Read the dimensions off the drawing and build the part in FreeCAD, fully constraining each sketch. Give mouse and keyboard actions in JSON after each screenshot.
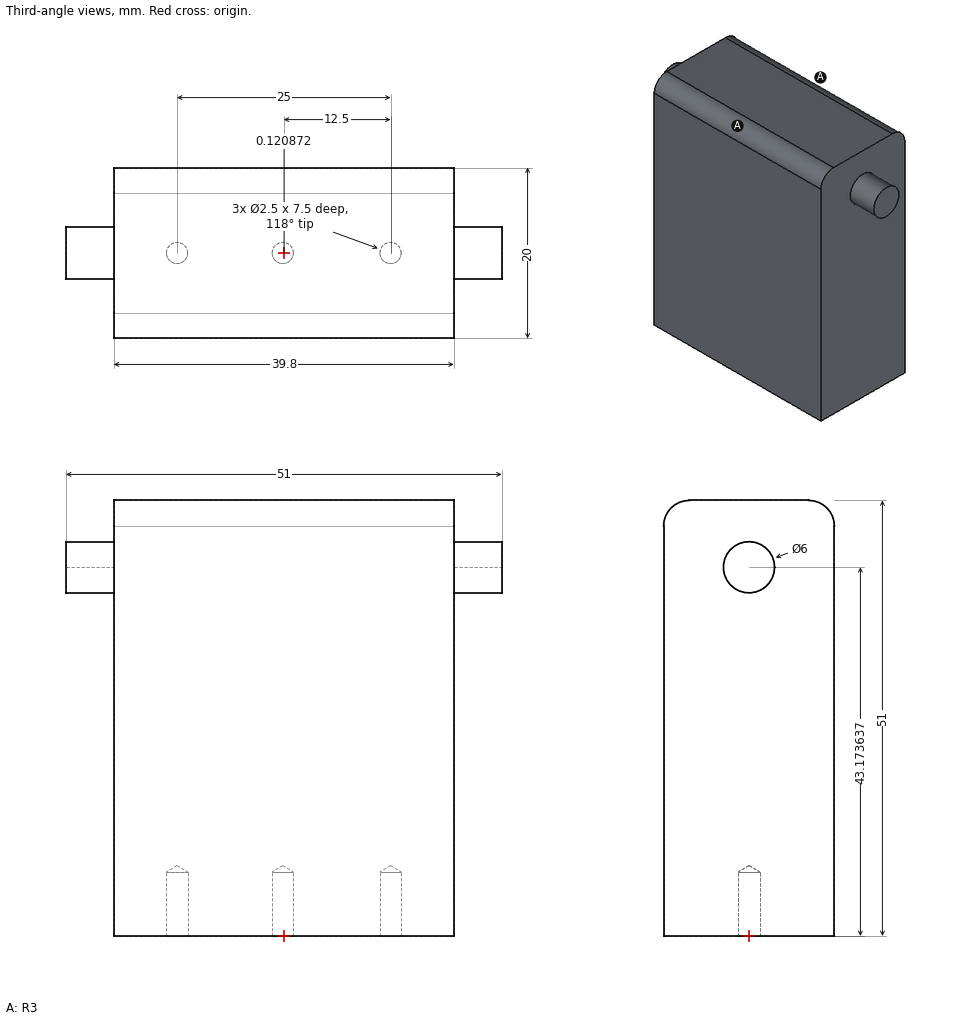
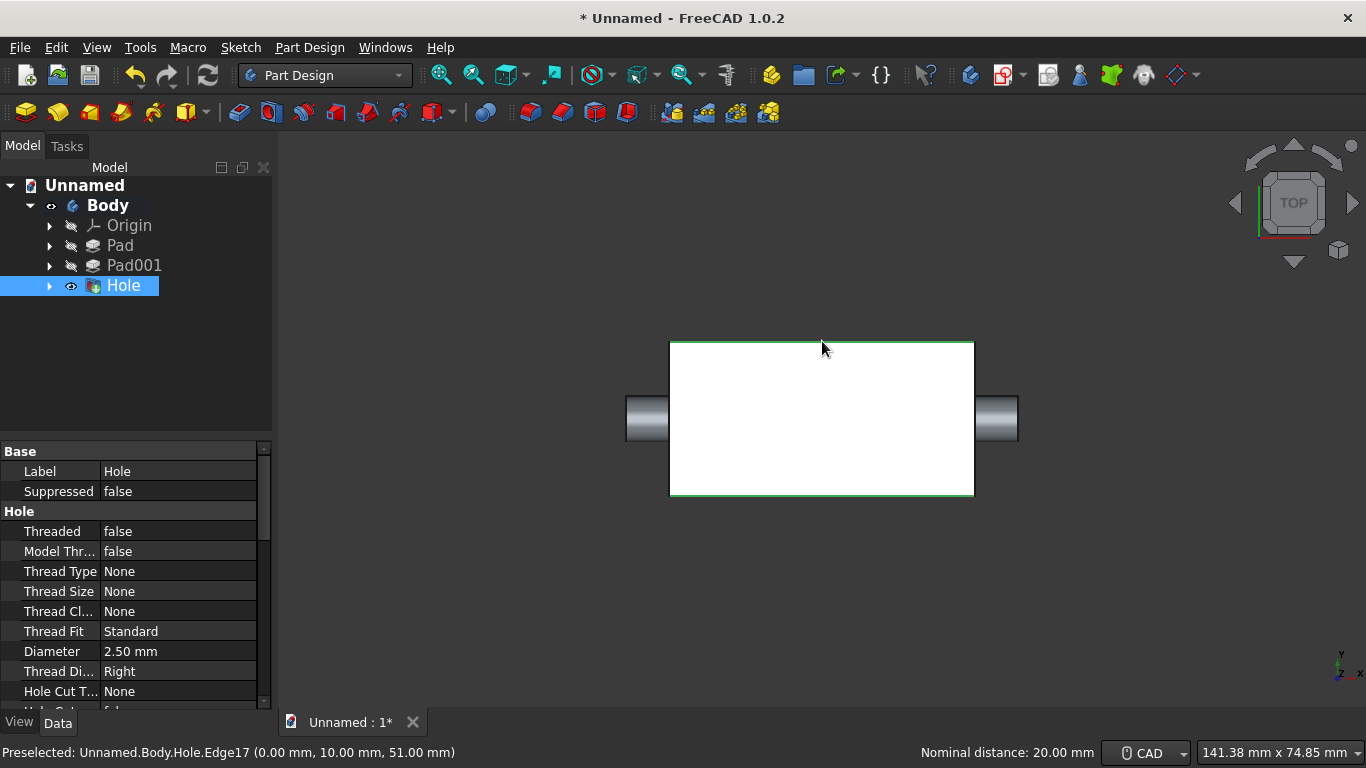
{"action": "left_click", "coordinate": [532, 112]}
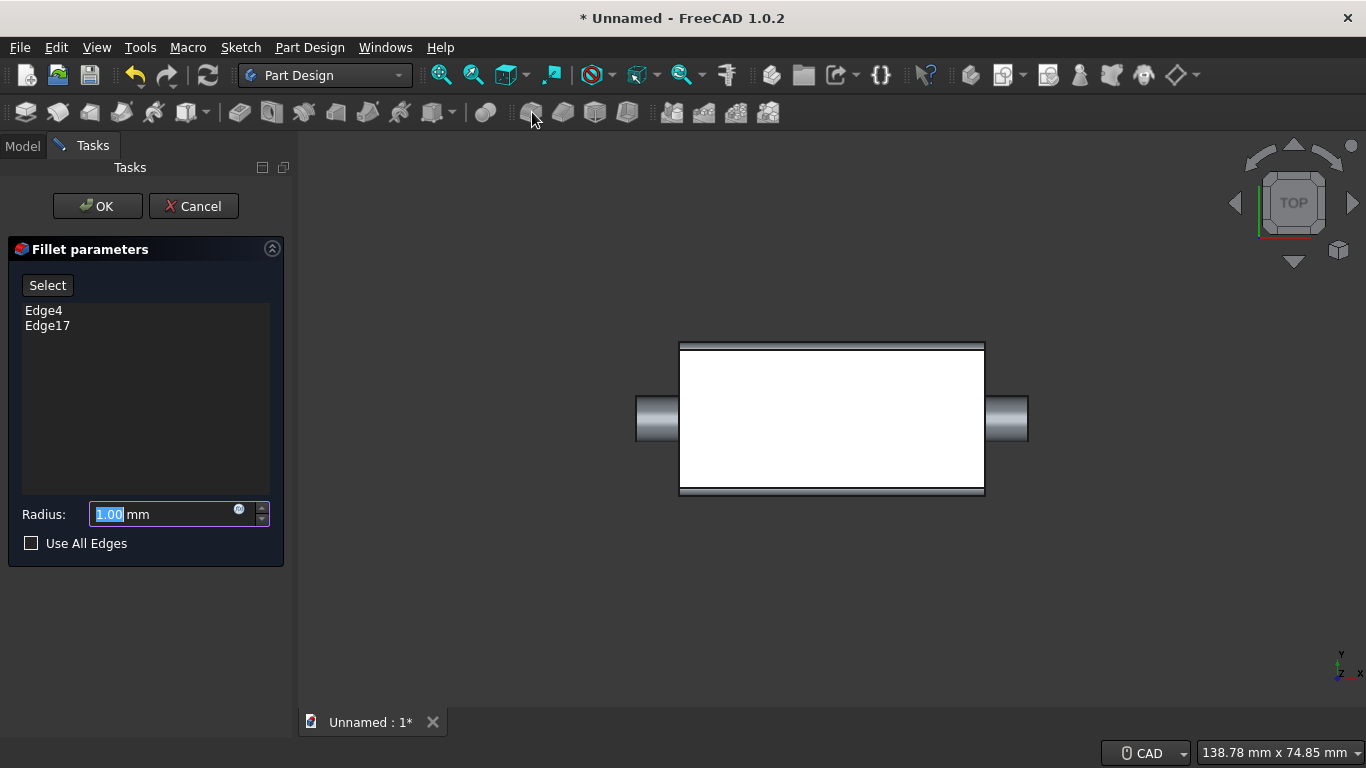
{"action": "type", "text": "3"}
{"action": "key", "text": "Tab"}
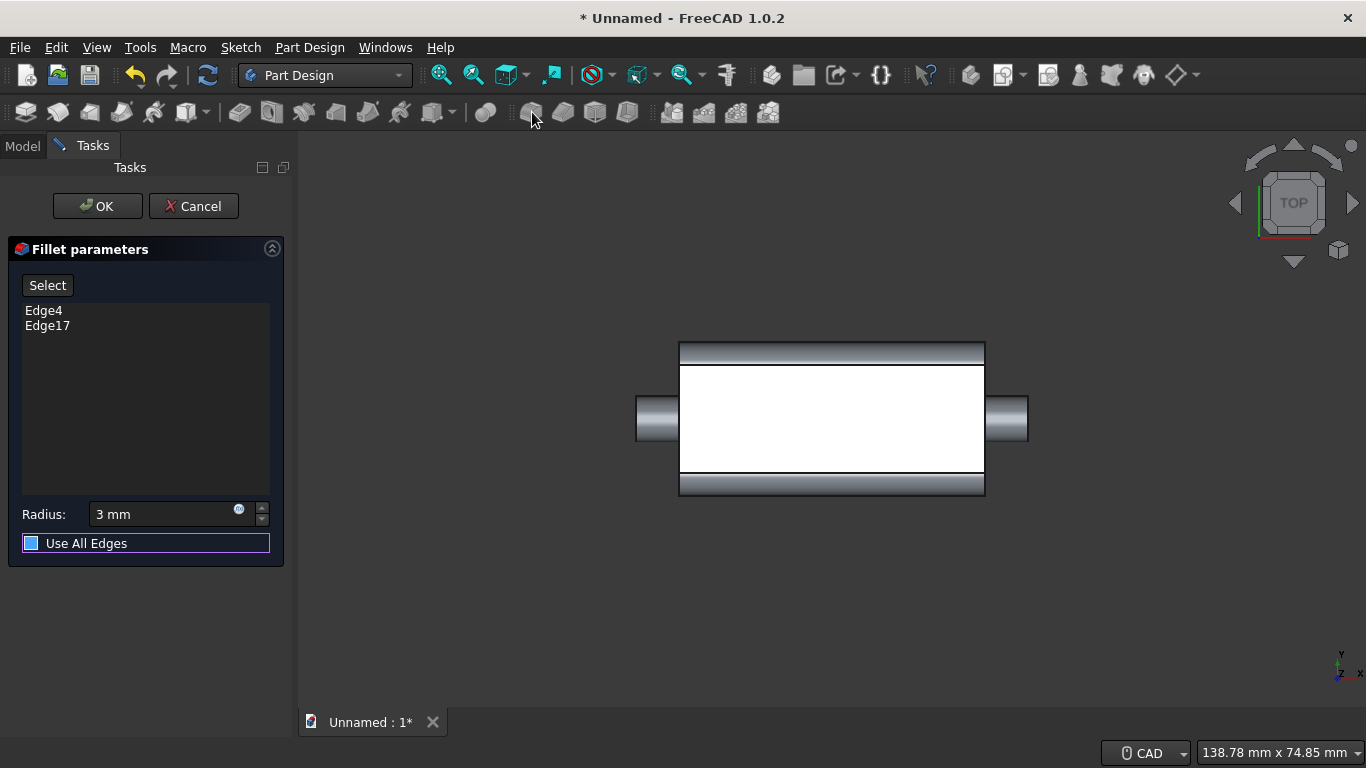
{"action": "left_click", "coordinate": [98, 206]}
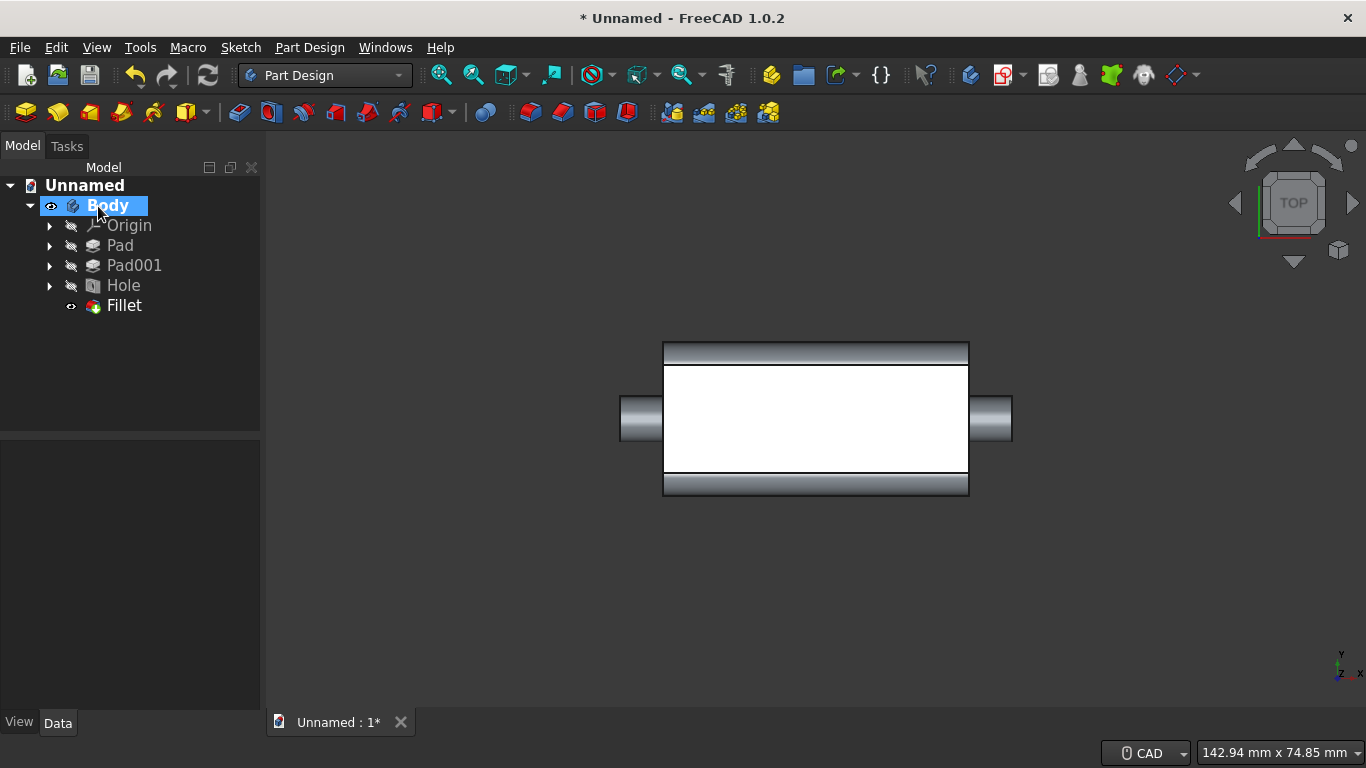
{"action": "key", "text": "0"}